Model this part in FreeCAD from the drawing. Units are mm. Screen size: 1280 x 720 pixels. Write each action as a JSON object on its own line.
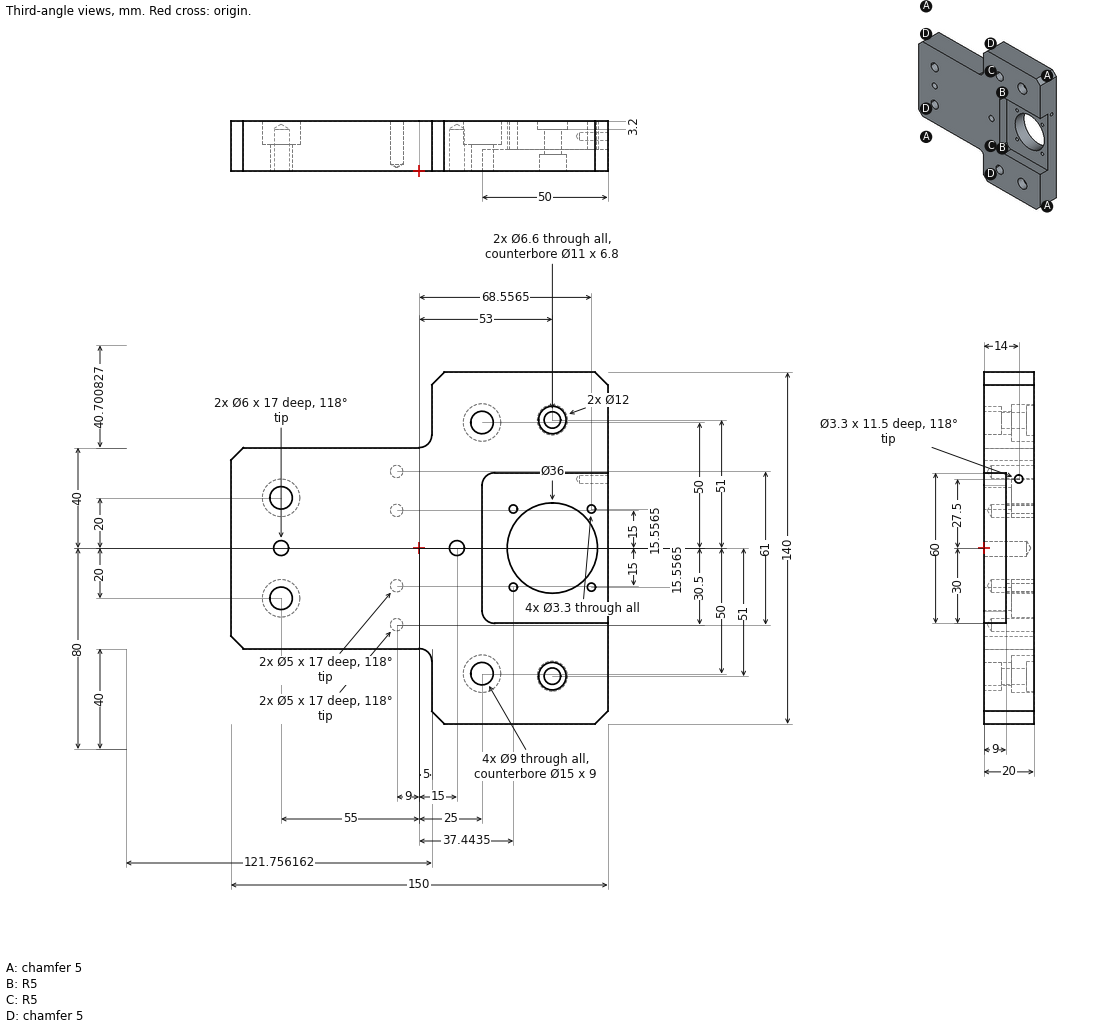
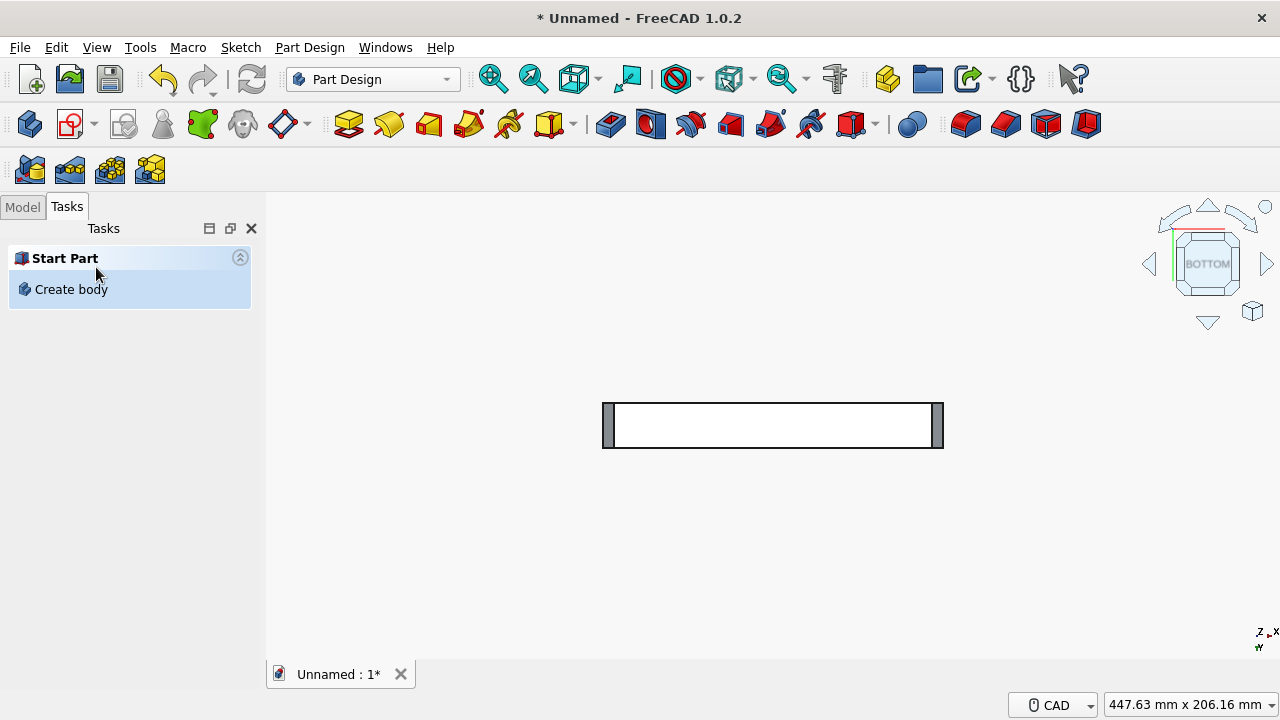
{"action": "left_click", "coordinate": [494, 80]}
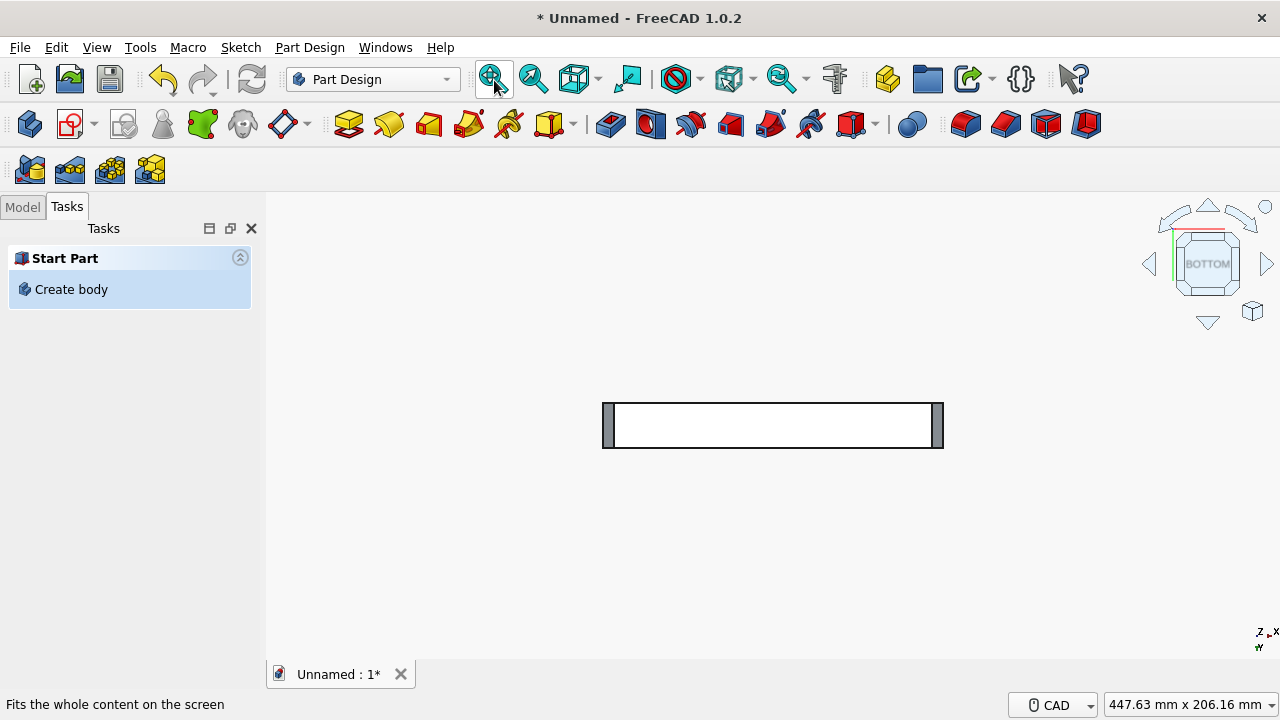
{"action": "key", "text": "4"}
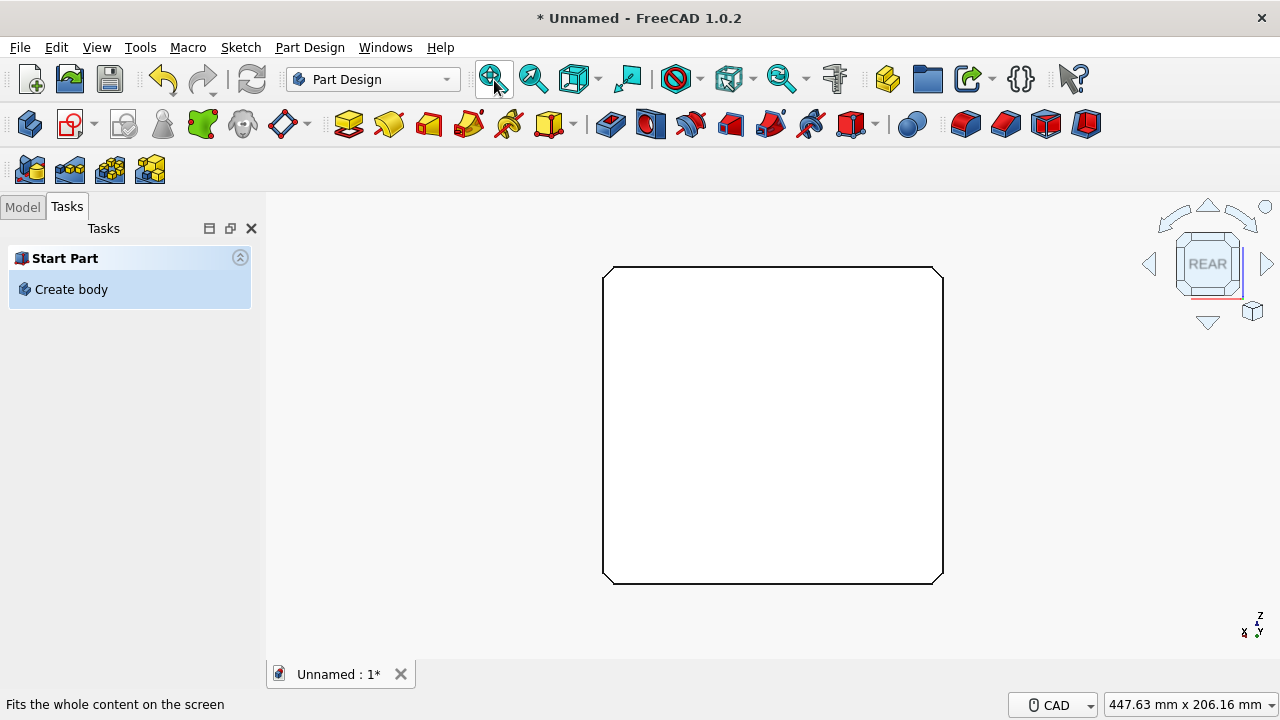
{"action": "left_click", "coordinate": [773, 424]}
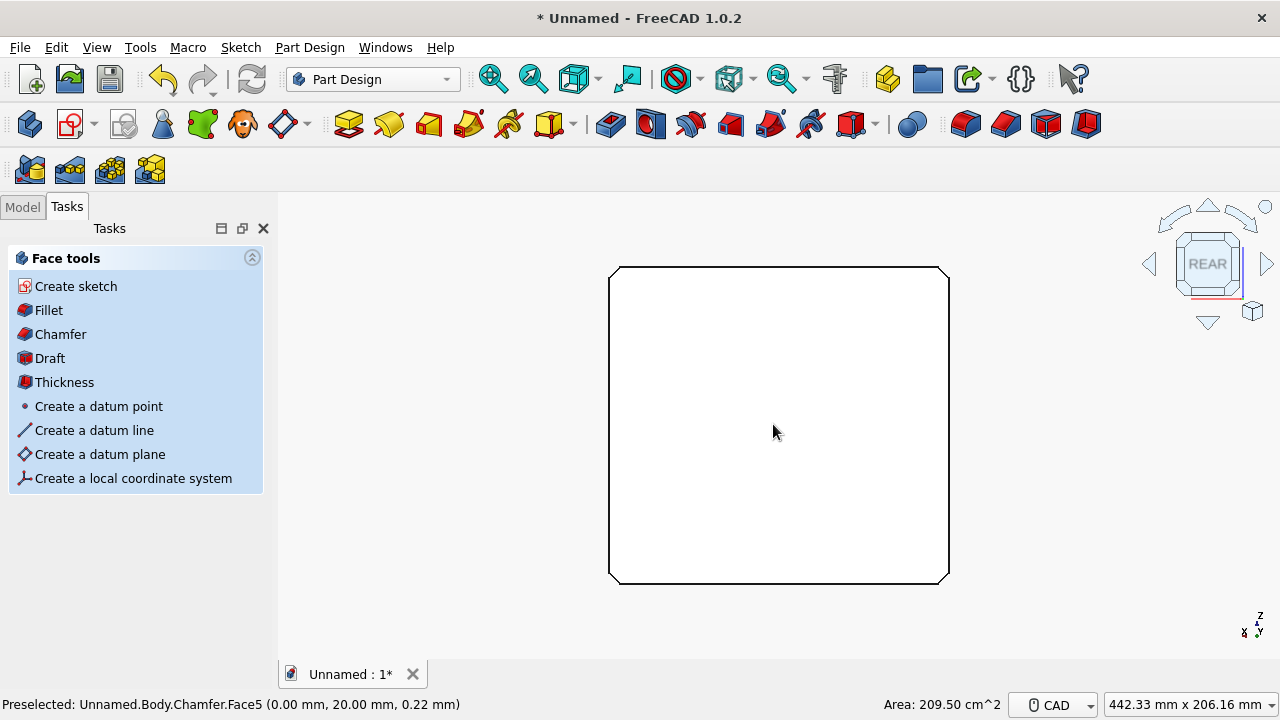
{"action": "left_click", "coordinate": [70, 124]}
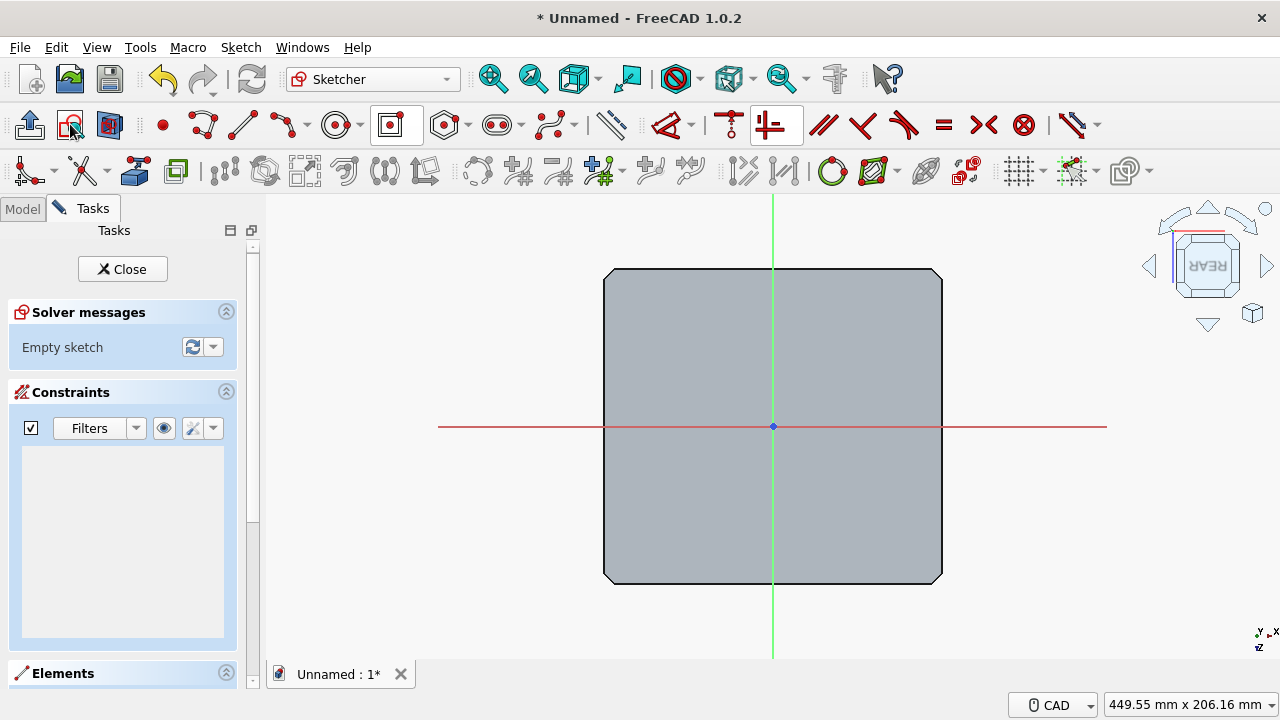
{"action": "left_click", "coordinate": [336, 126]}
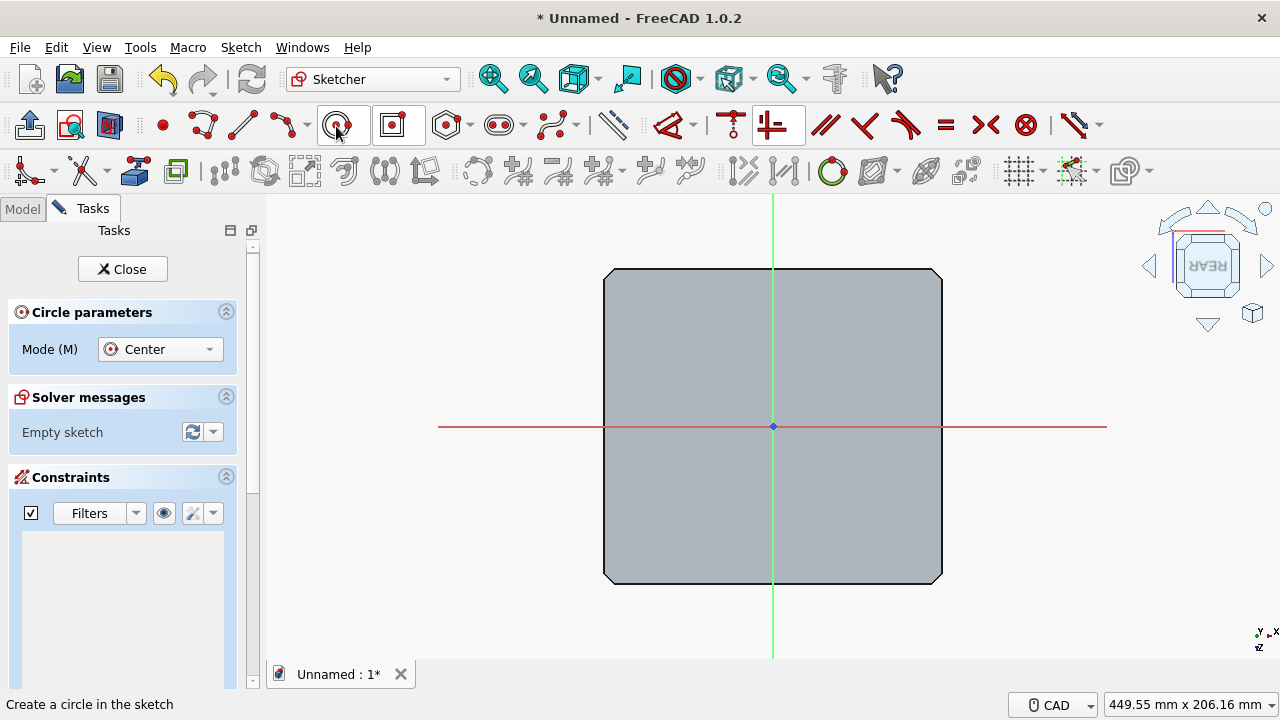
{"action": "scroll", "coordinate": [893, 542], "scroll_direction": "up", "scroll_amount": 3}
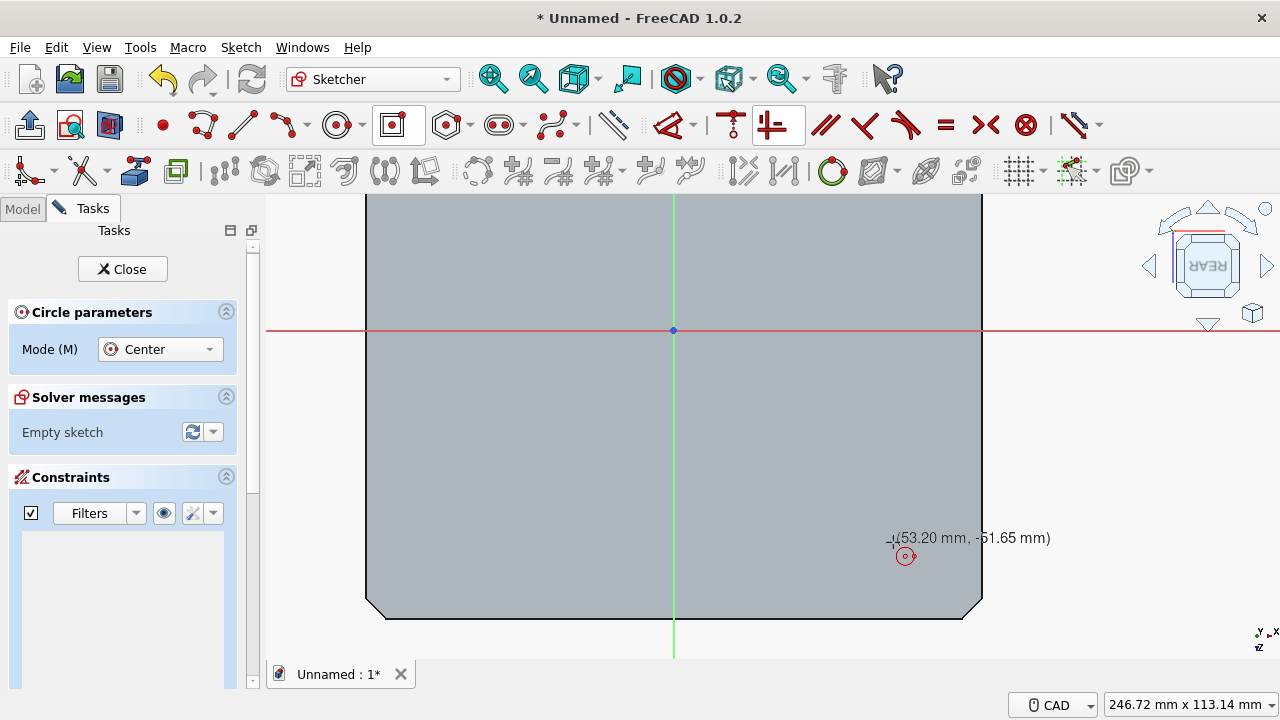
{"action": "left_click", "coordinate": [892, 541]}
{"action": "left_click", "coordinate": [909, 523]}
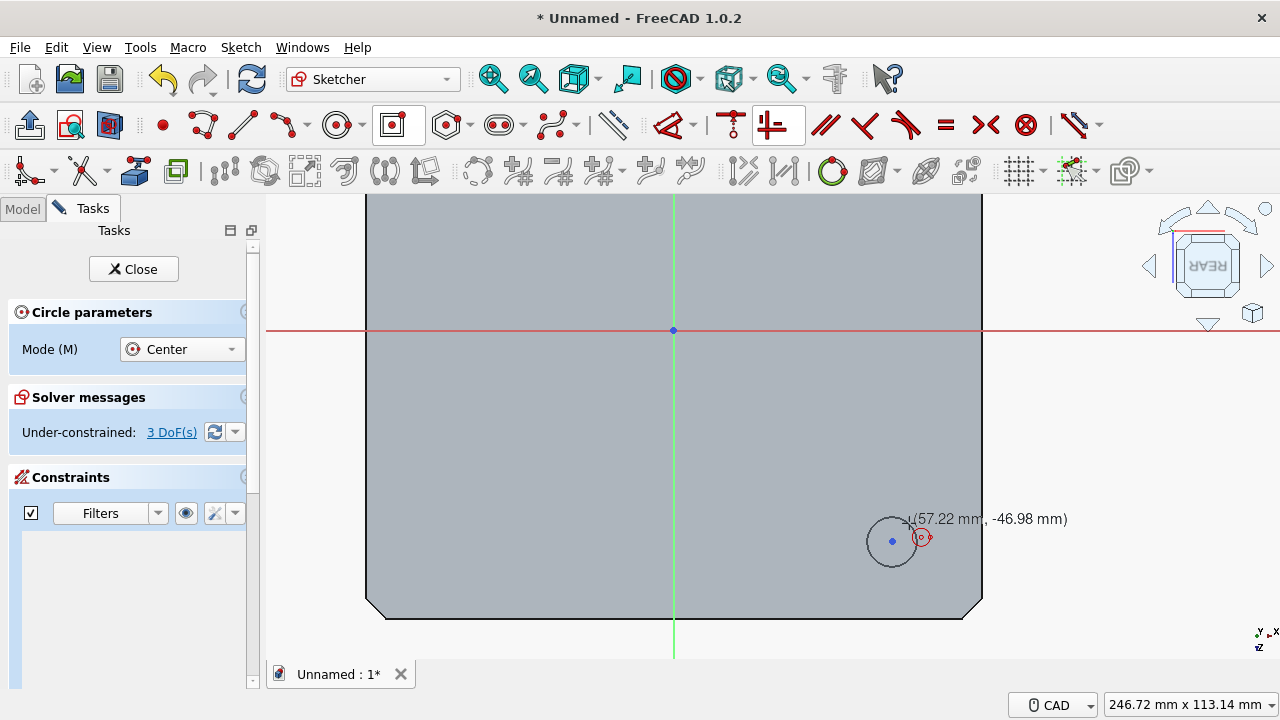
{"action": "scroll", "coordinate": [520, 621], "scroll_direction": "down", "scroll_amount": 2}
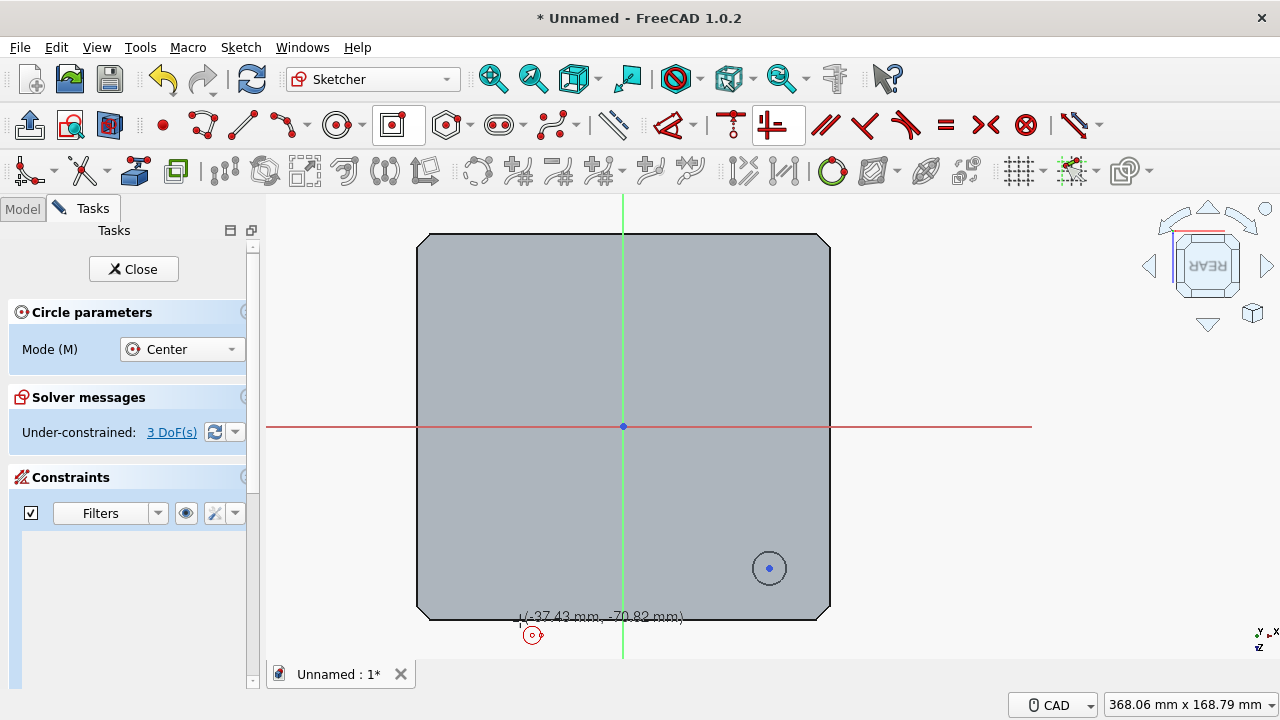
{"action": "scroll", "coordinate": [769, 286], "scroll_direction": "up", "scroll_amount": 2}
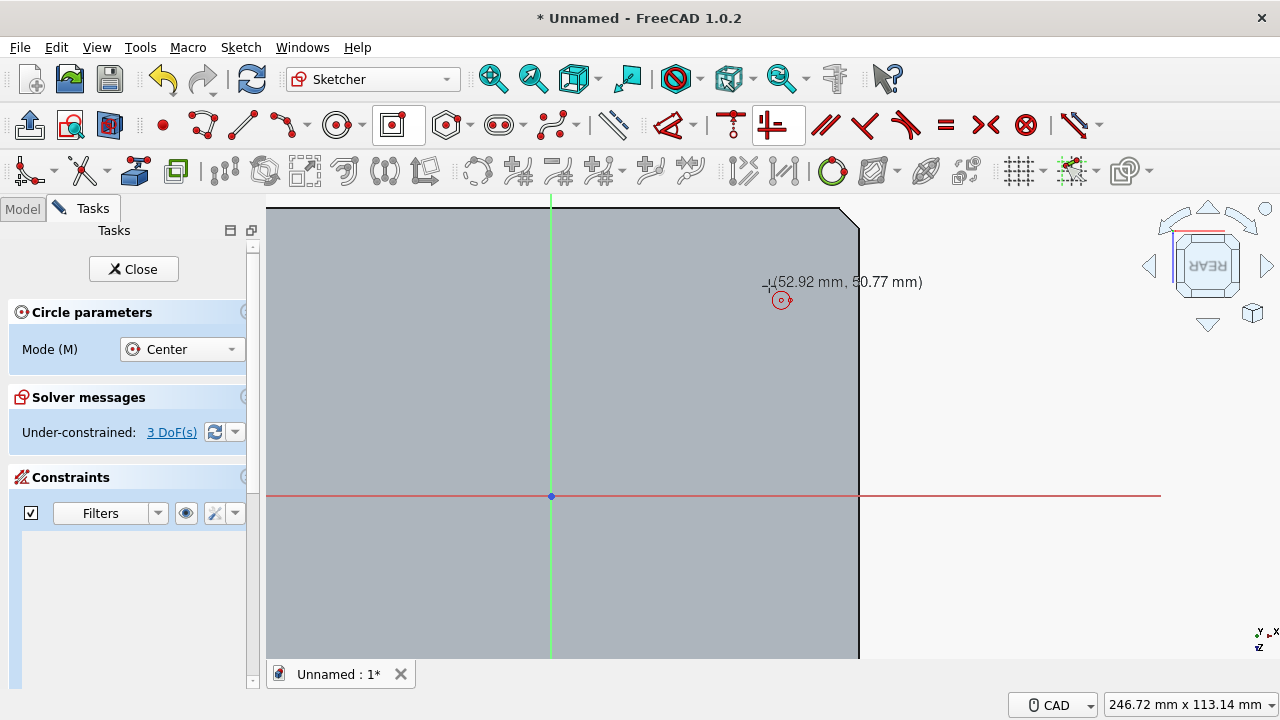
{"action": "left_click", "coordinate": [769, 286]}
{"action": "left_click", "coordinate": [787, 269]}
{"action": "key", "text": "Escape"}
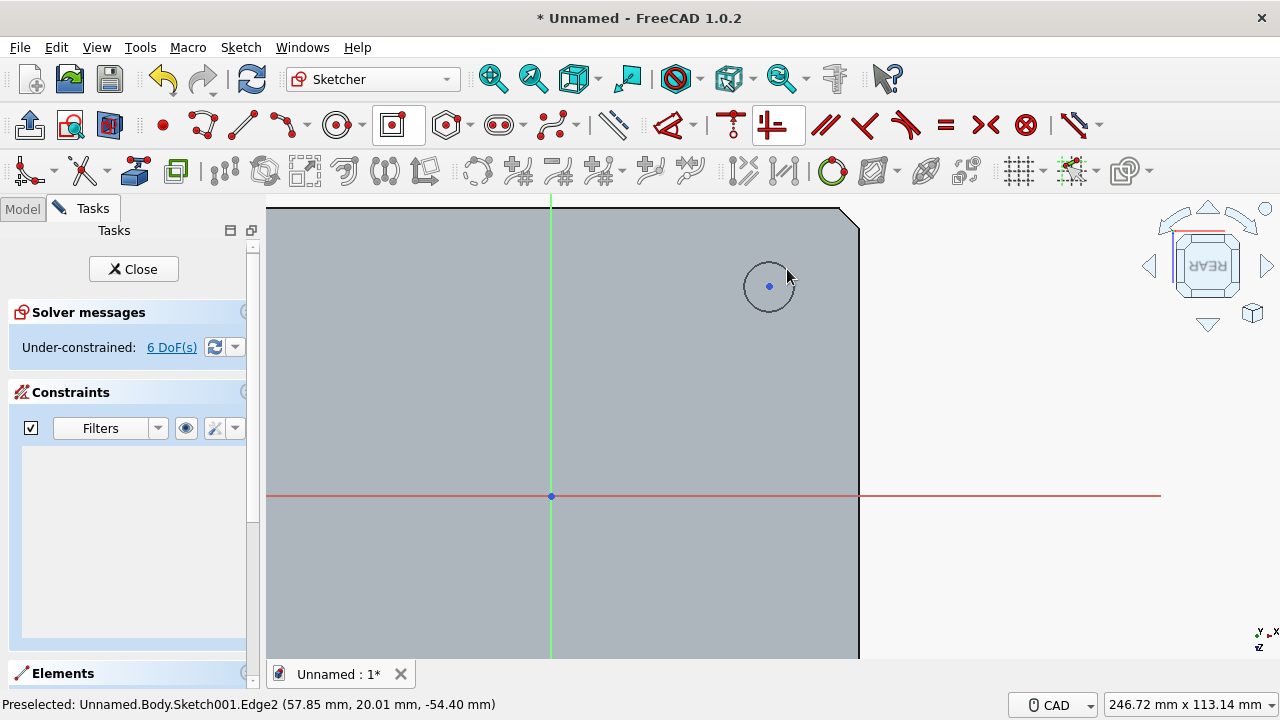
{"action": "scroll", "coordinate": [770, 285], "scroll_direction": "down", "scroll_amount": 2}